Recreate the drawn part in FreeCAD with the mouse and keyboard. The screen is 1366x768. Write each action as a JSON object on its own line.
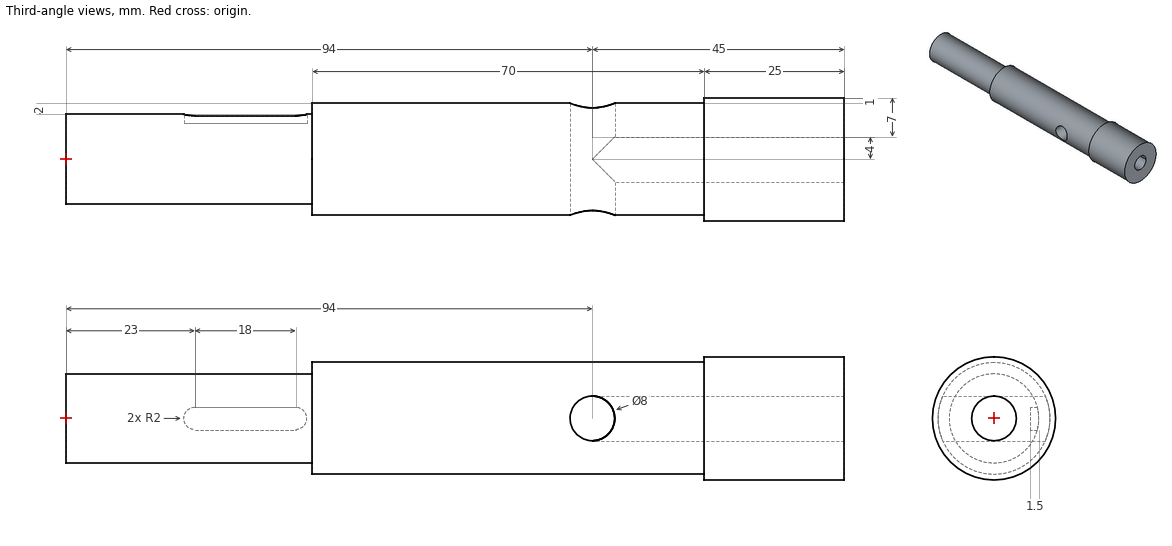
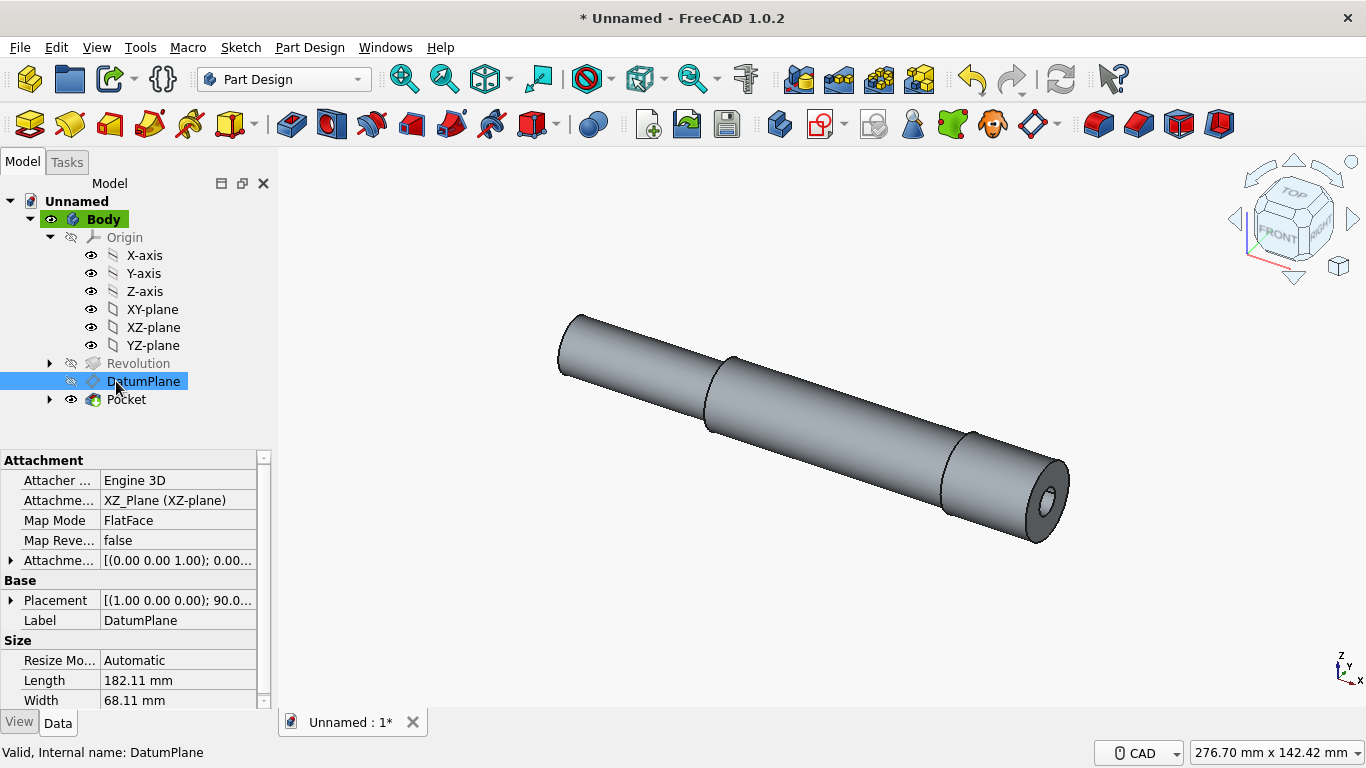
{"action": "left_click", "coordinate": [318, 667]}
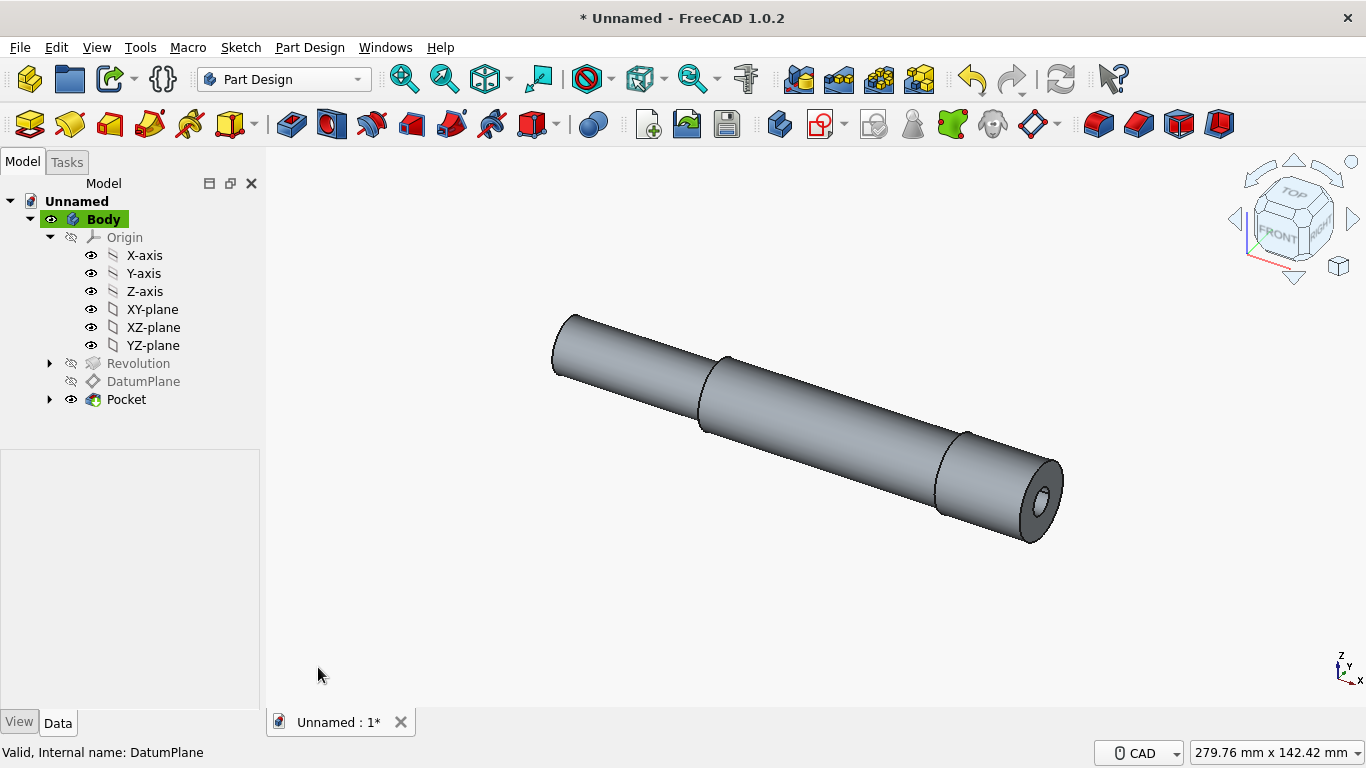
{"action": "left_click", "coordinate": [820, 124]}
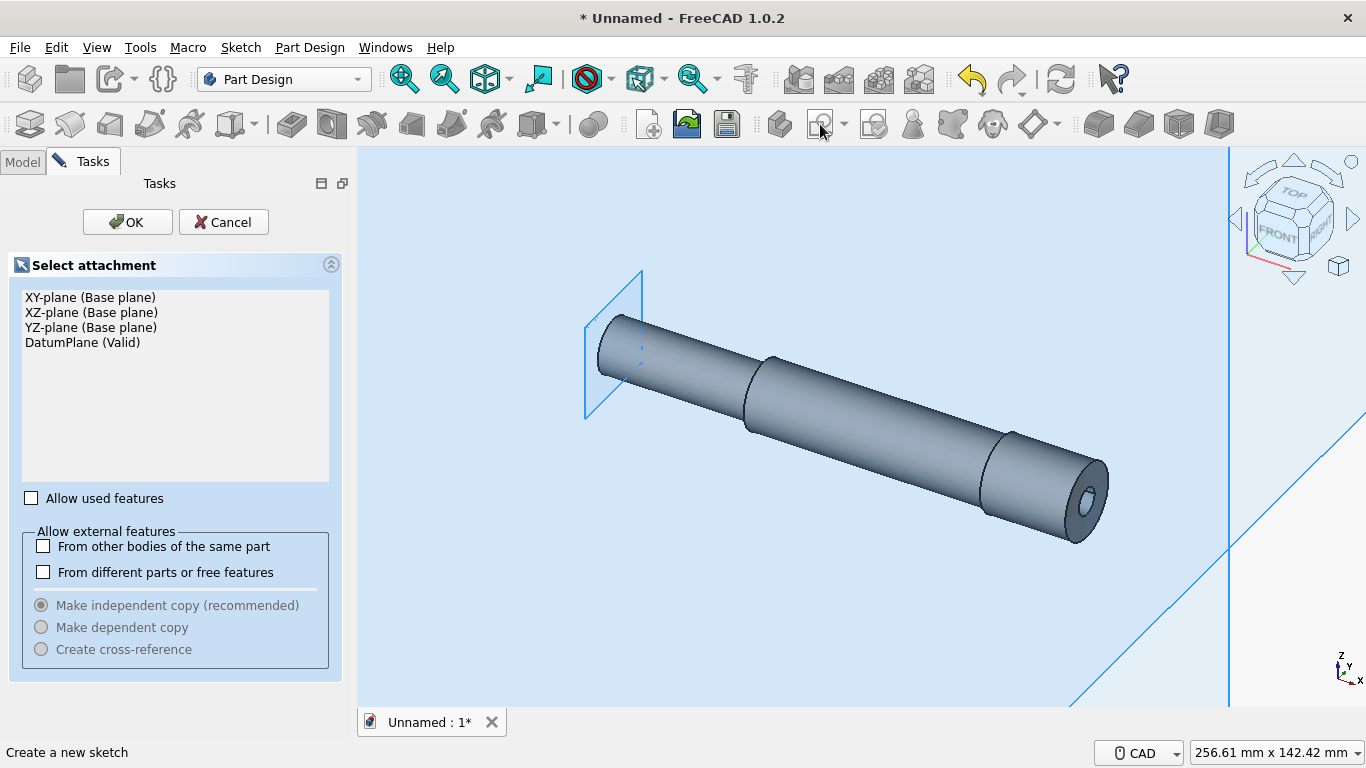
{"action": "left_click", "coordinate": [82, 312]}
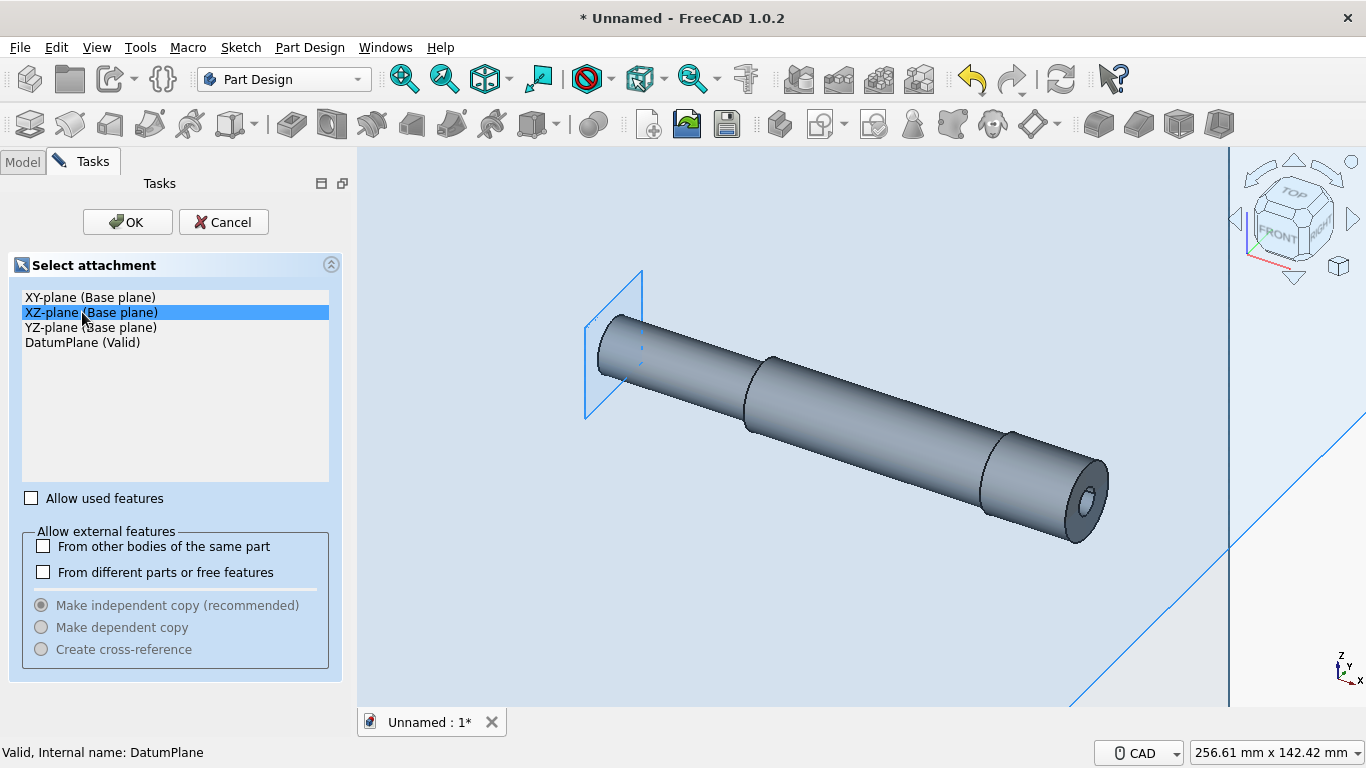
{"action": "left_click", "coordinate": [128, 222]}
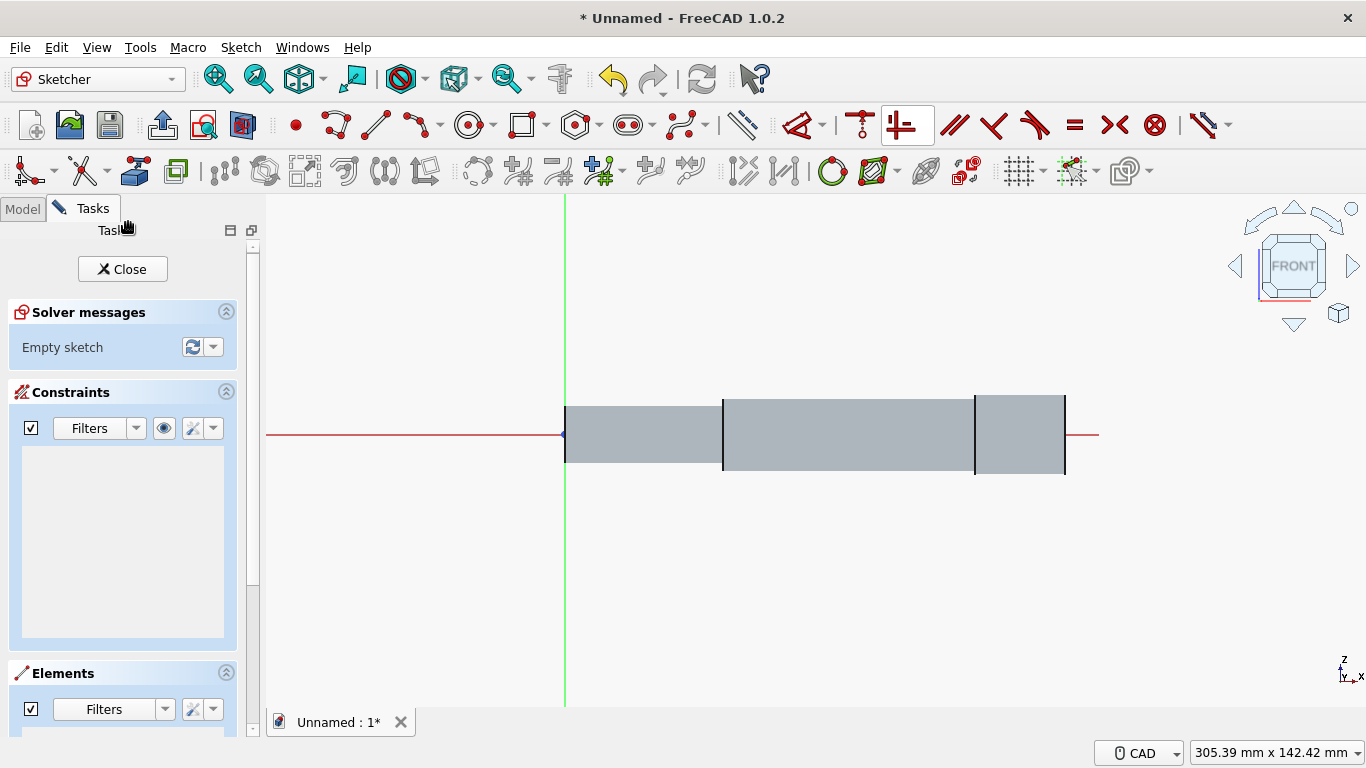
{"action": "key", "text": "q s"}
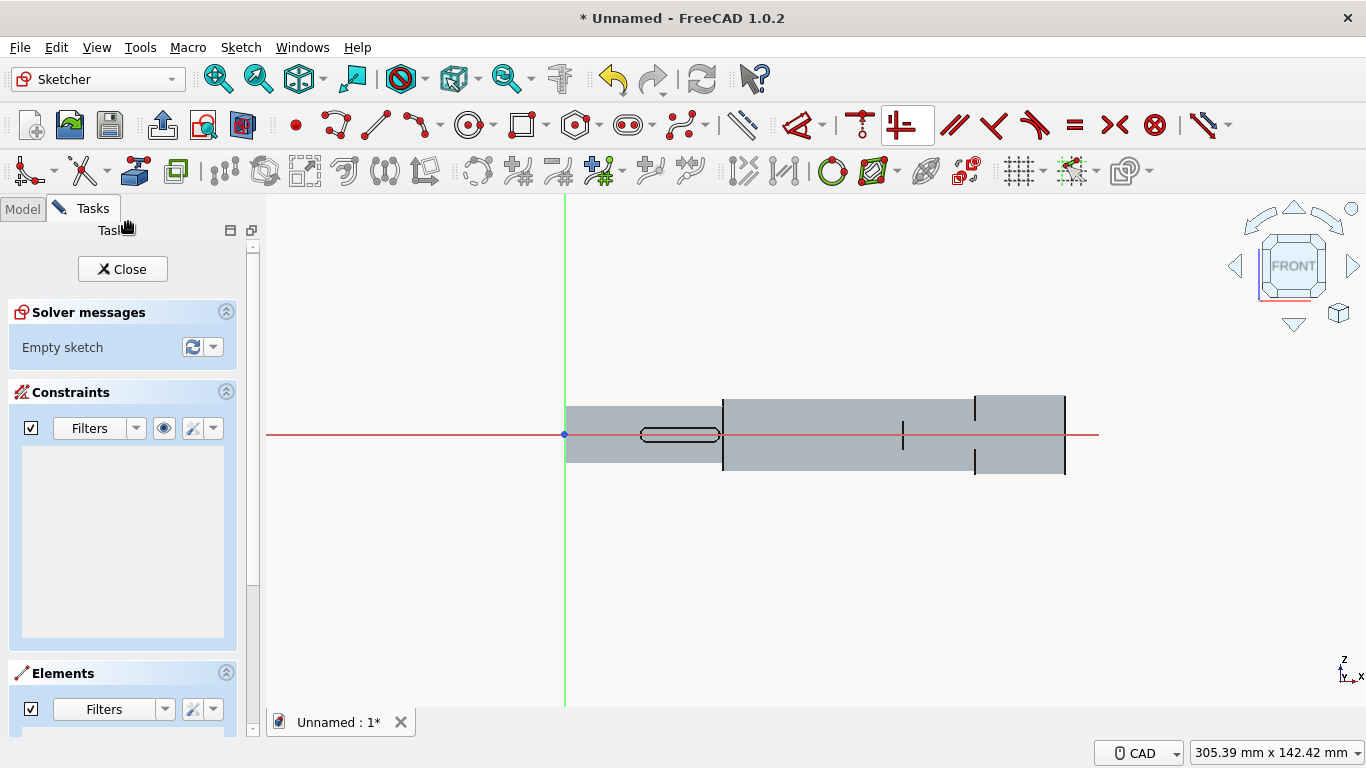
{"action": "scroll", "coordinate": [919, 433], "scroll_direction": "up", "scroll_amount": 12}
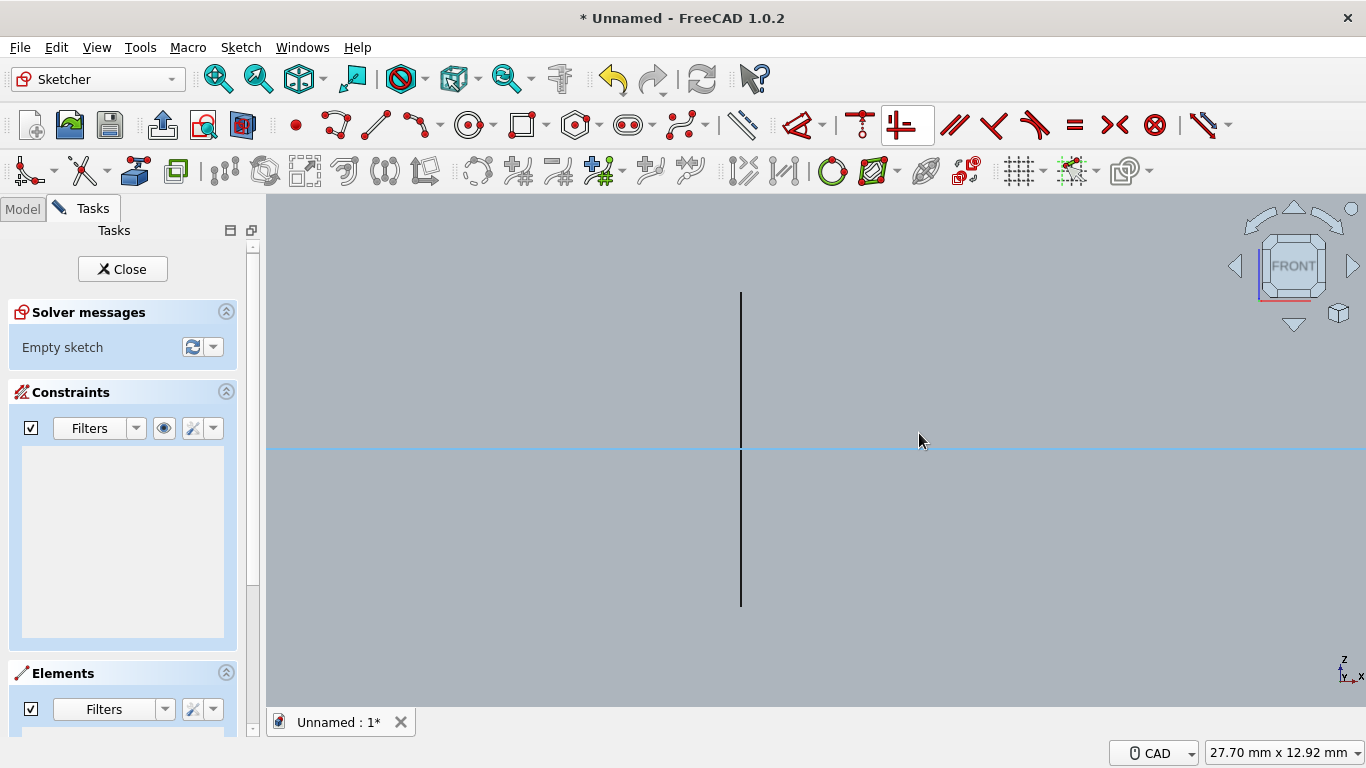
{"action": "key", "text": "g c"}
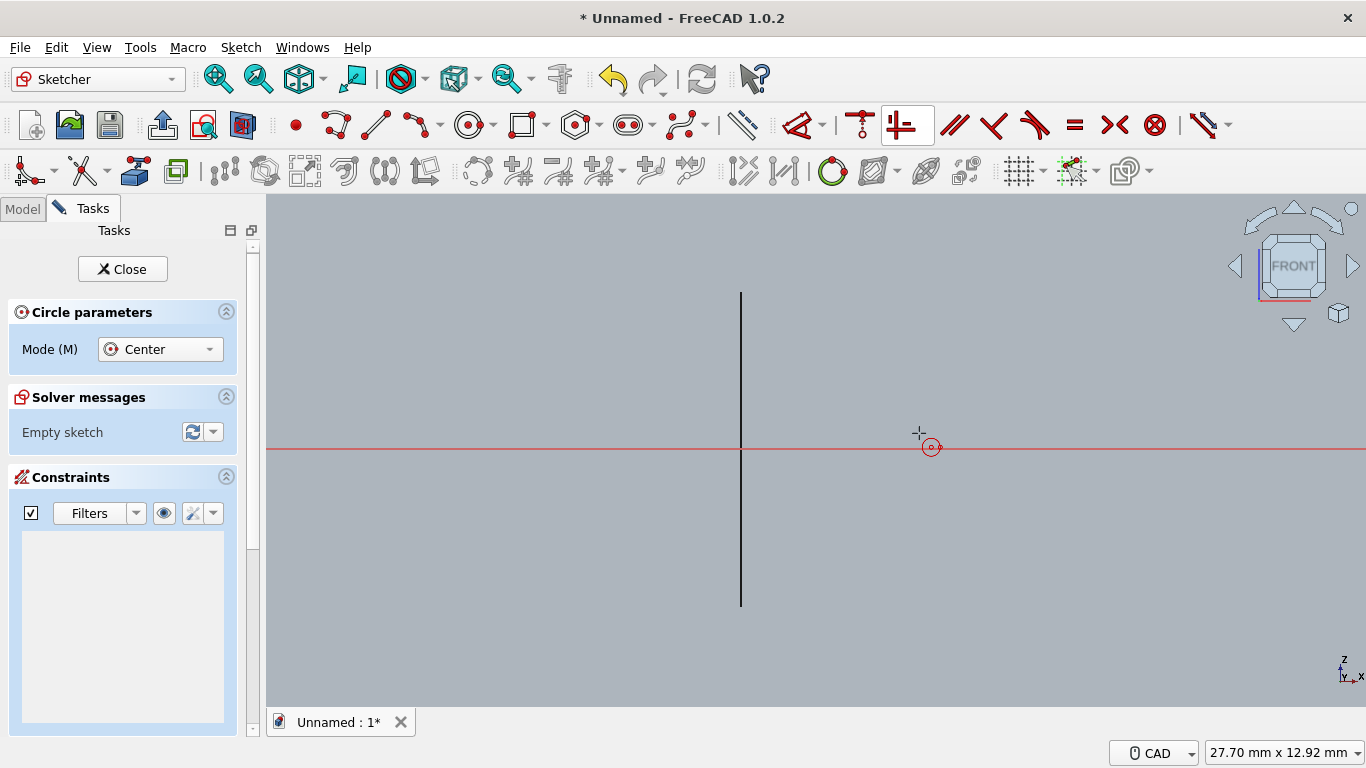
{"action": "left_click", "coordinate": [741, 449]}
{"action": "mouse_move", "coordinate": [853, 337]}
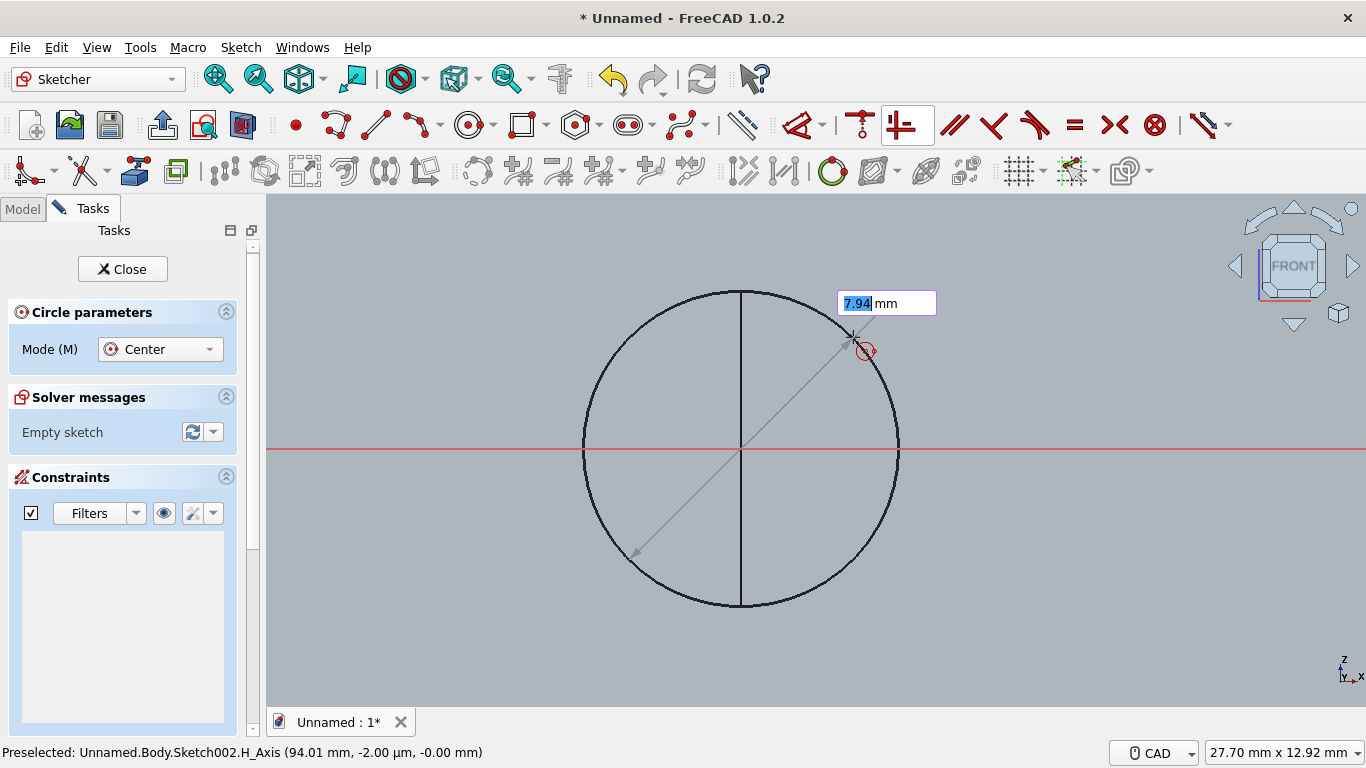
{"action": "type", "text": "8"}
{"action": "key", "text": "Return"}
{"action": "key", "text": "Escape"}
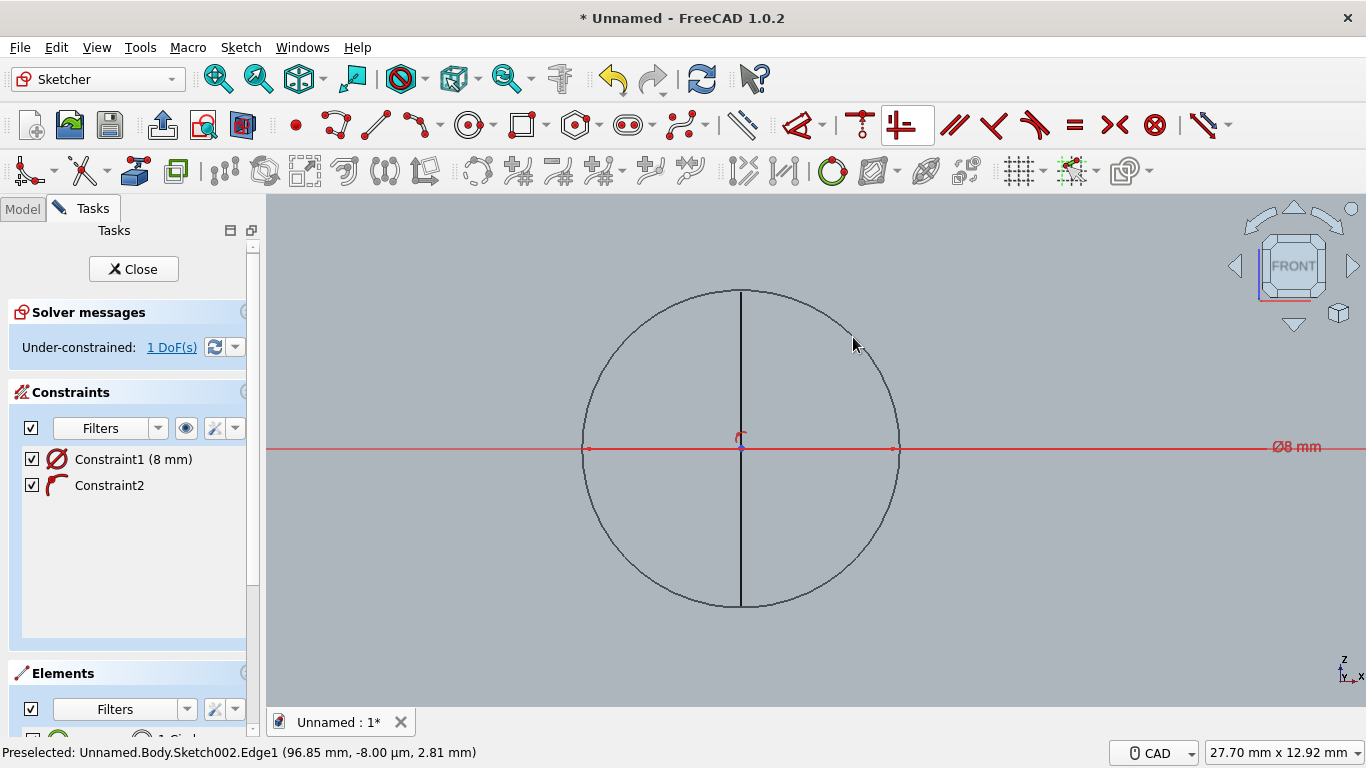
{"action": "key", "text": "d"}